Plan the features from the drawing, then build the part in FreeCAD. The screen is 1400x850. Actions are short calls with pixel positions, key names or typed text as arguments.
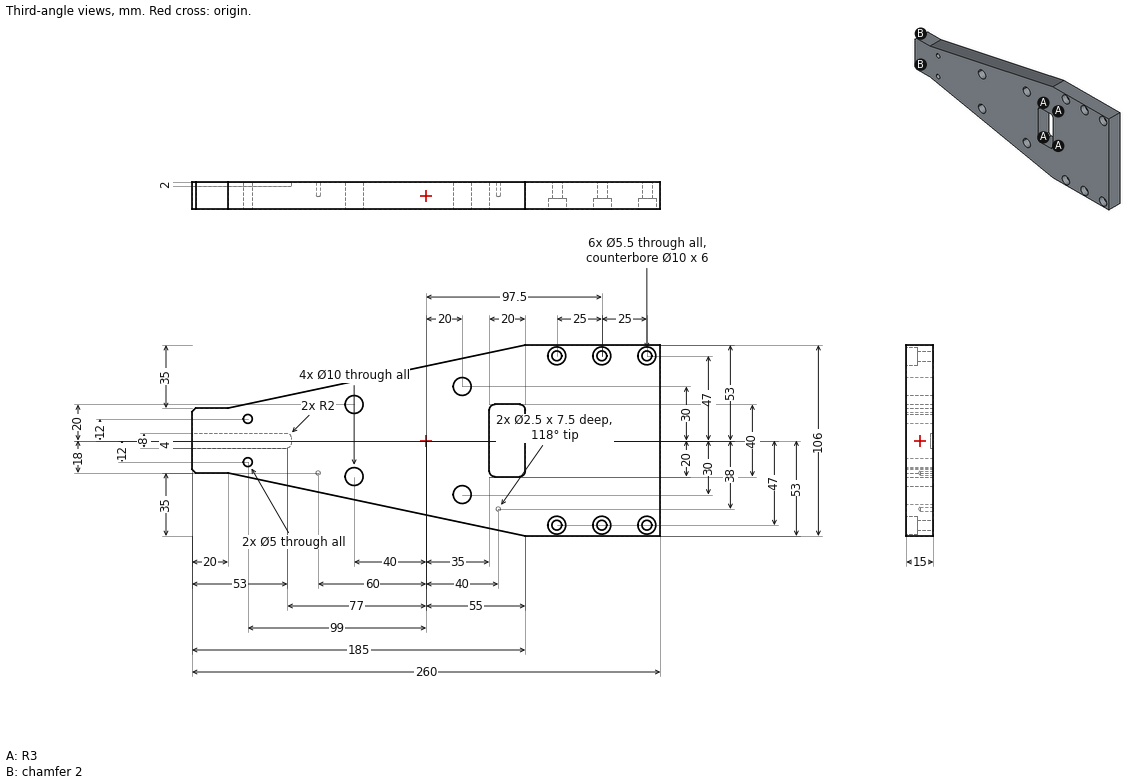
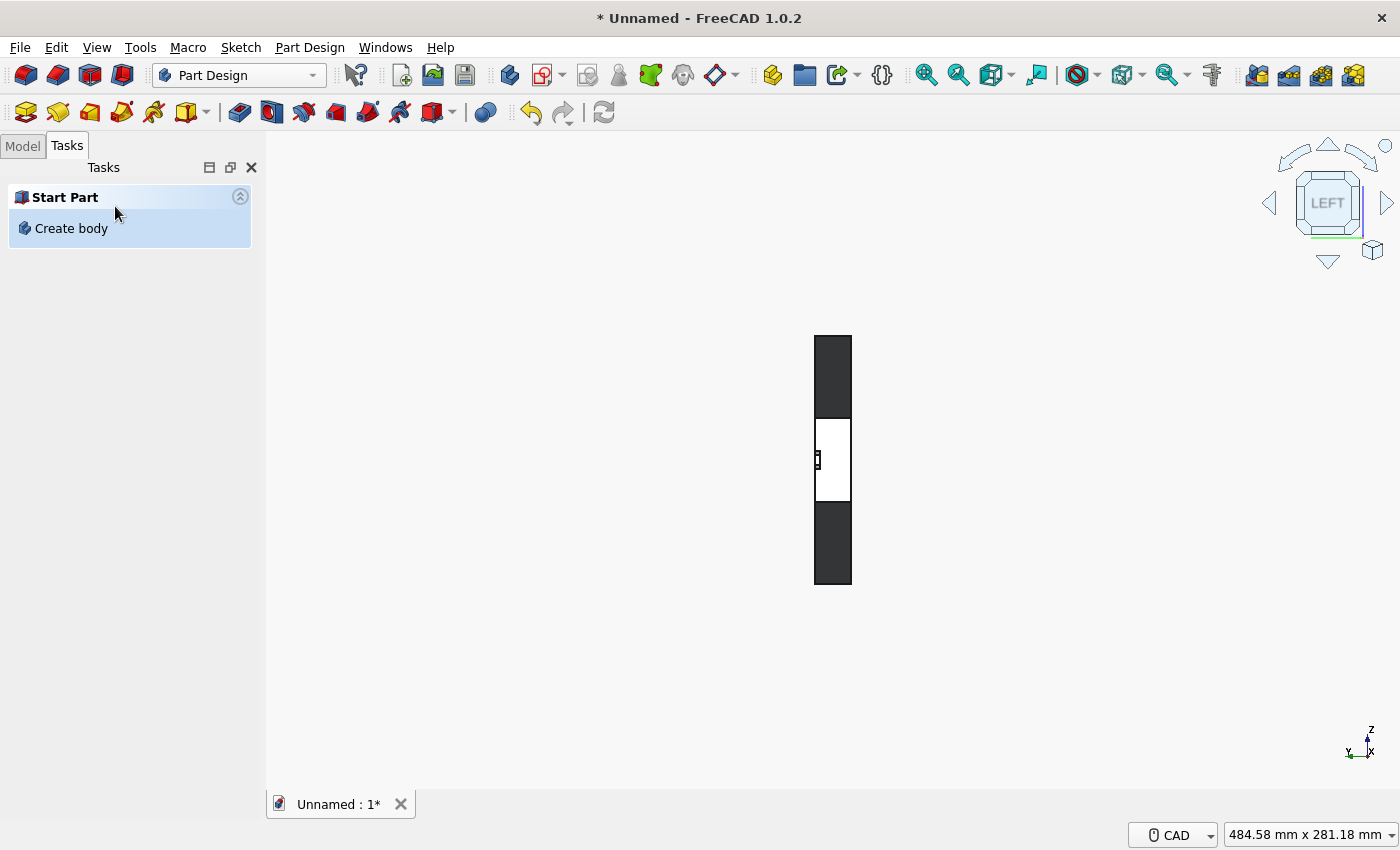
key(v)
key(3)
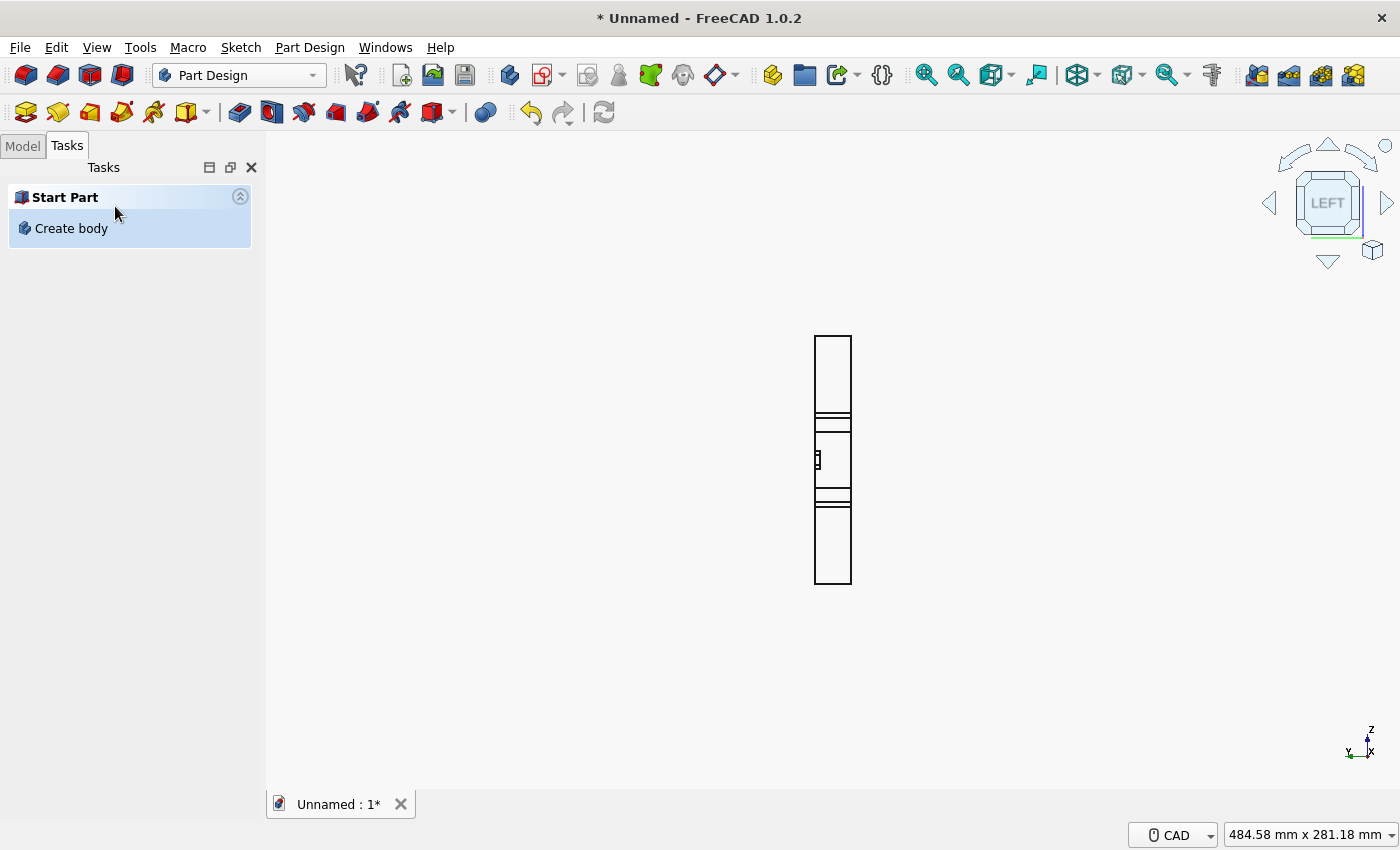
key(0)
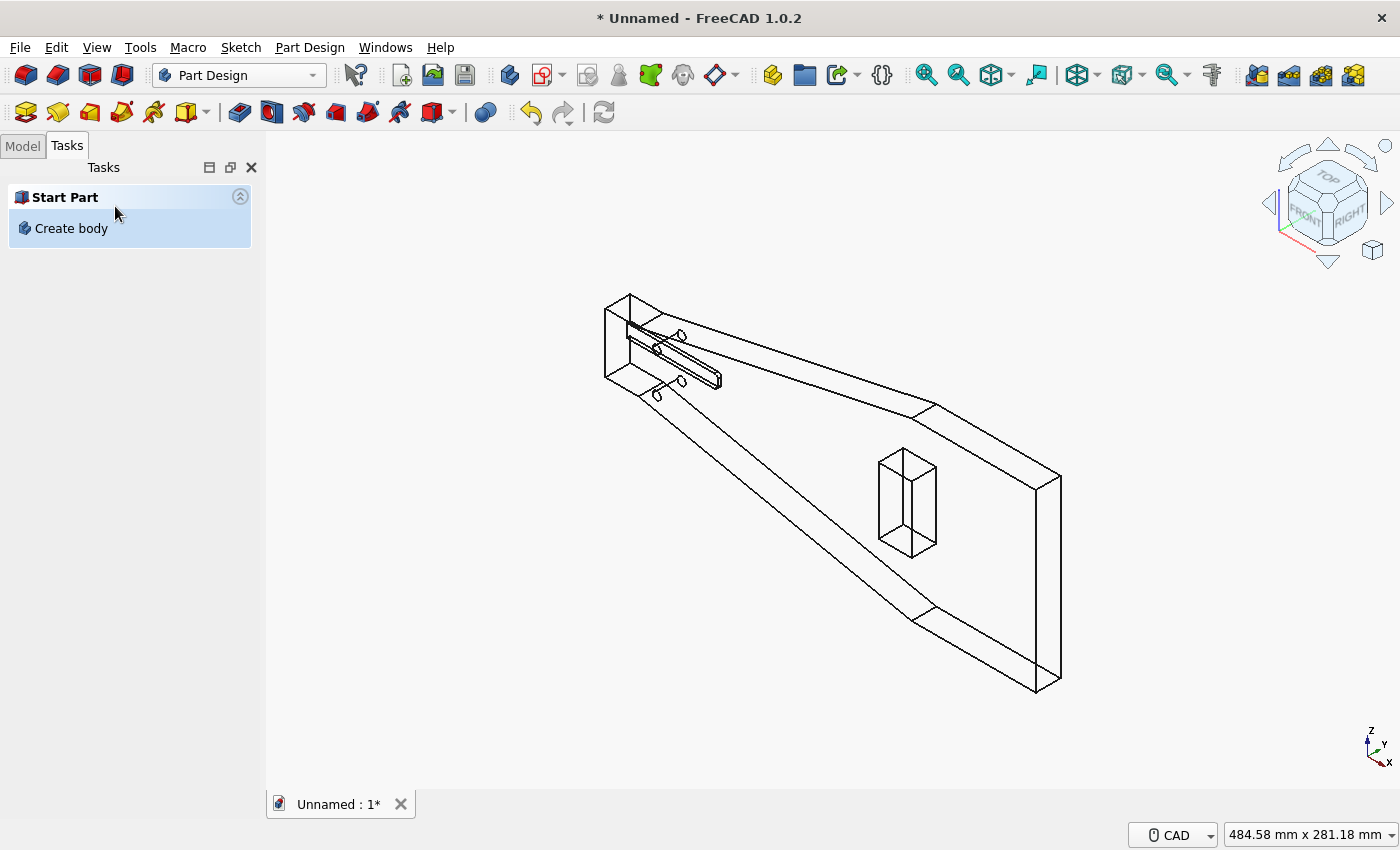
click(924, 550)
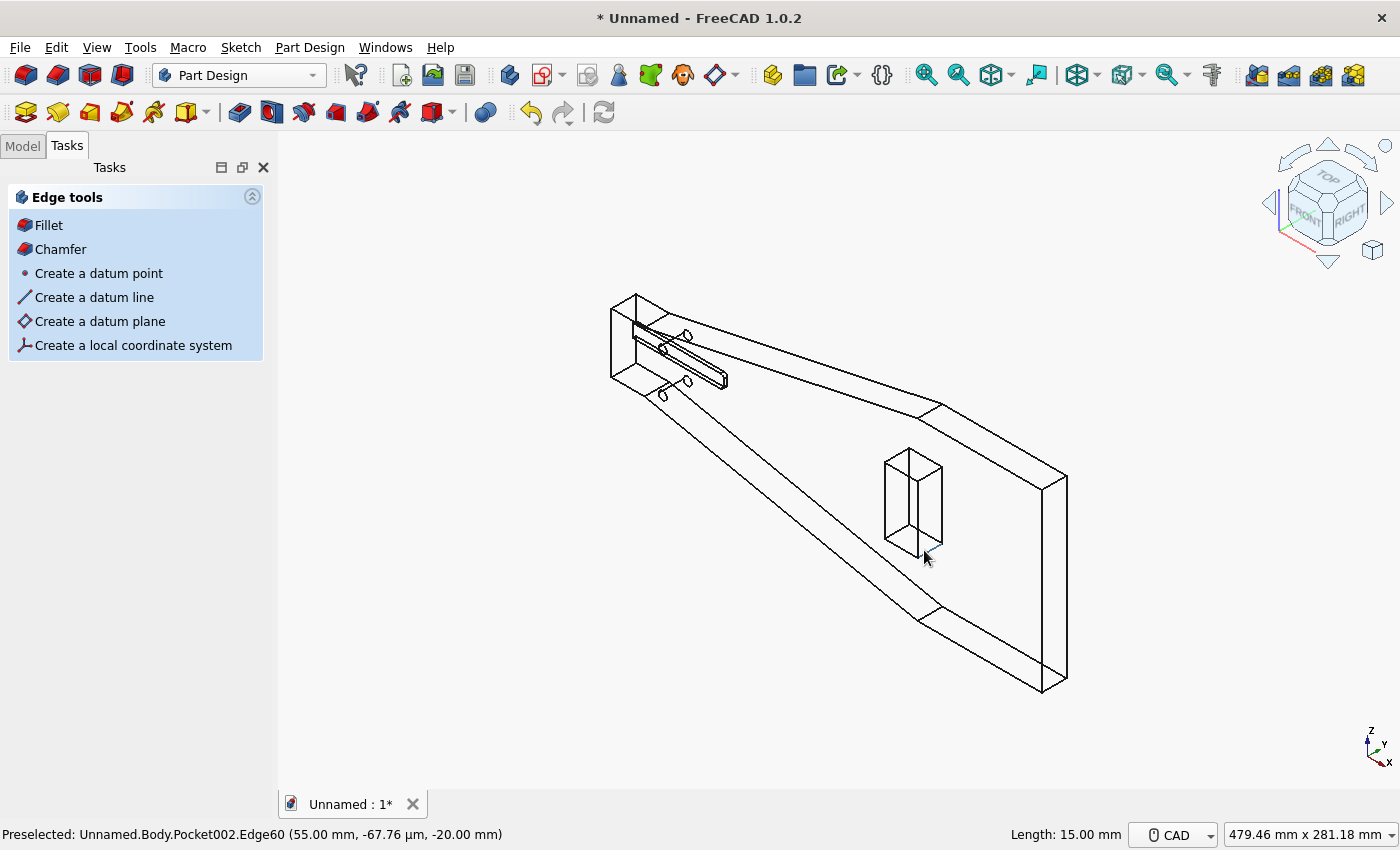
click(930, 473, ctrl)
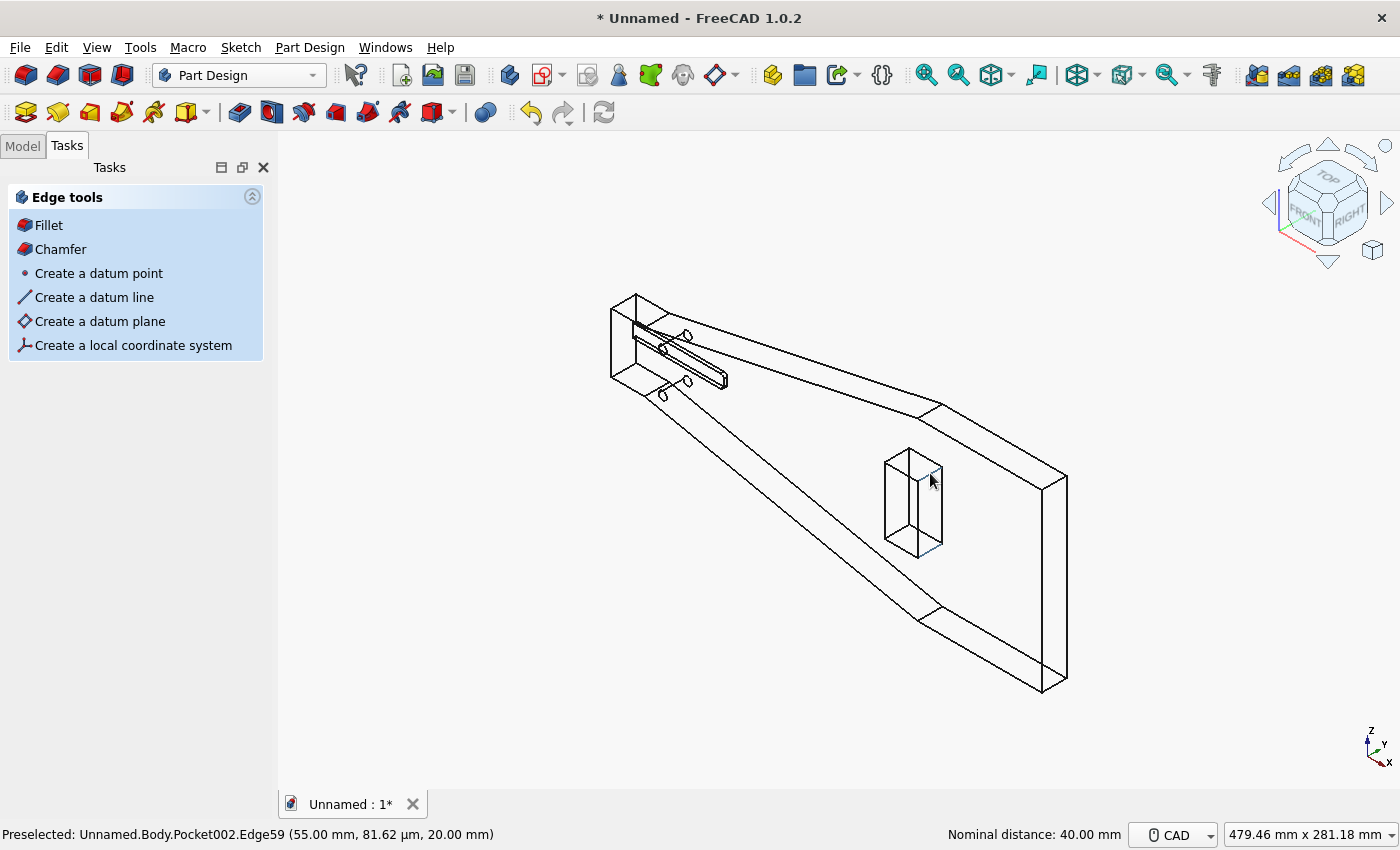
click(897, 454, ctrl)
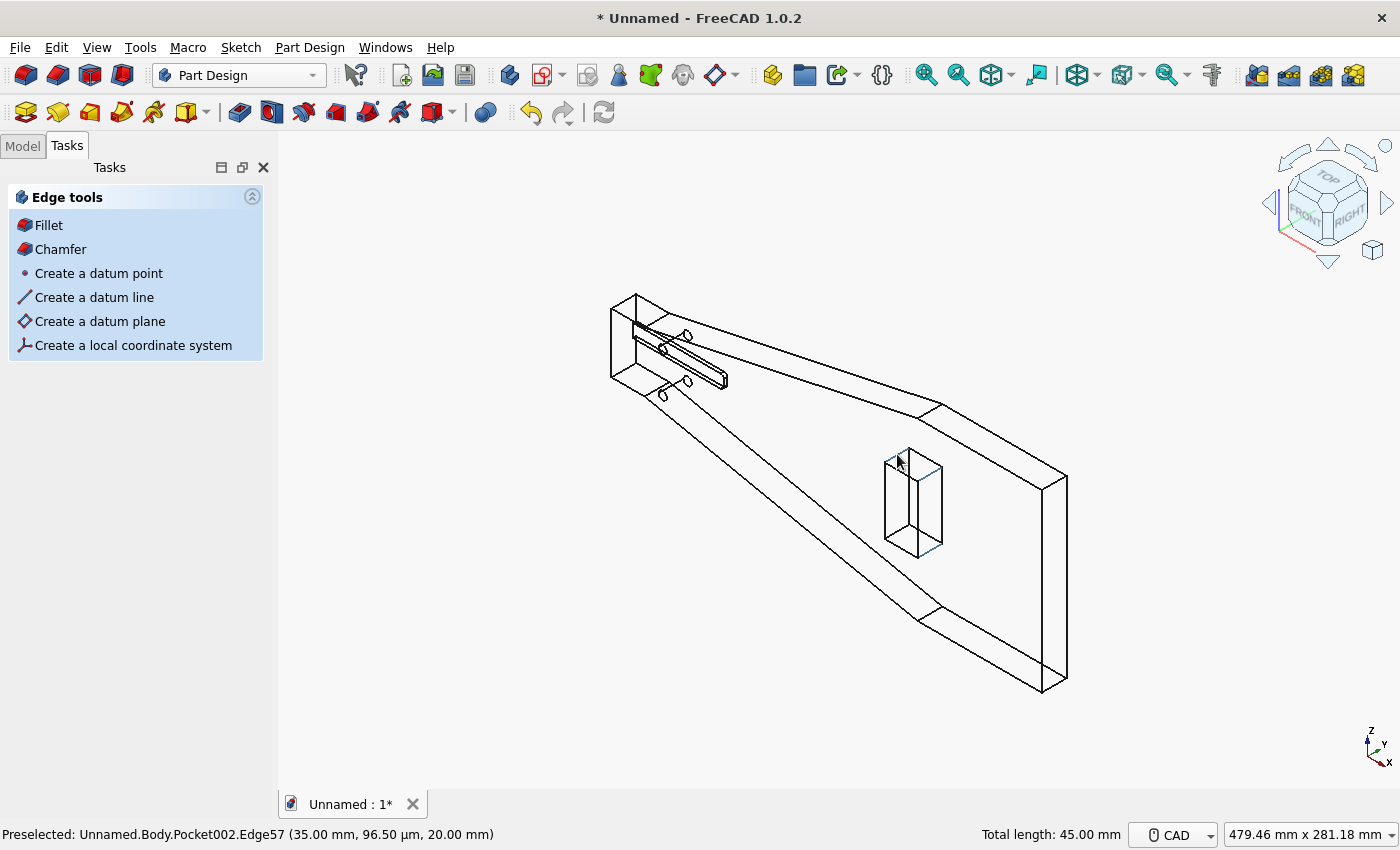
click(897, 531, ctrl)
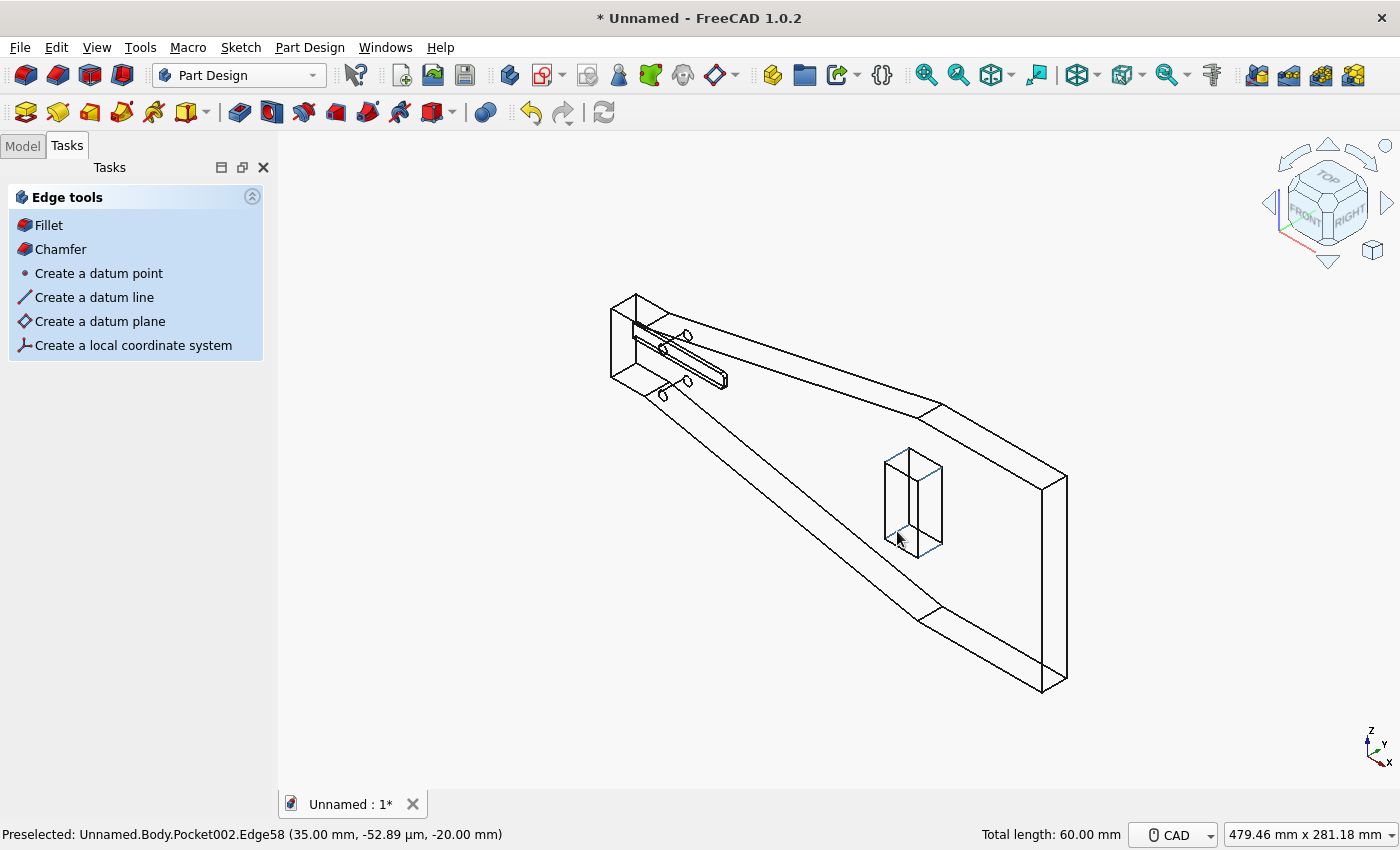
key(v)
key(1)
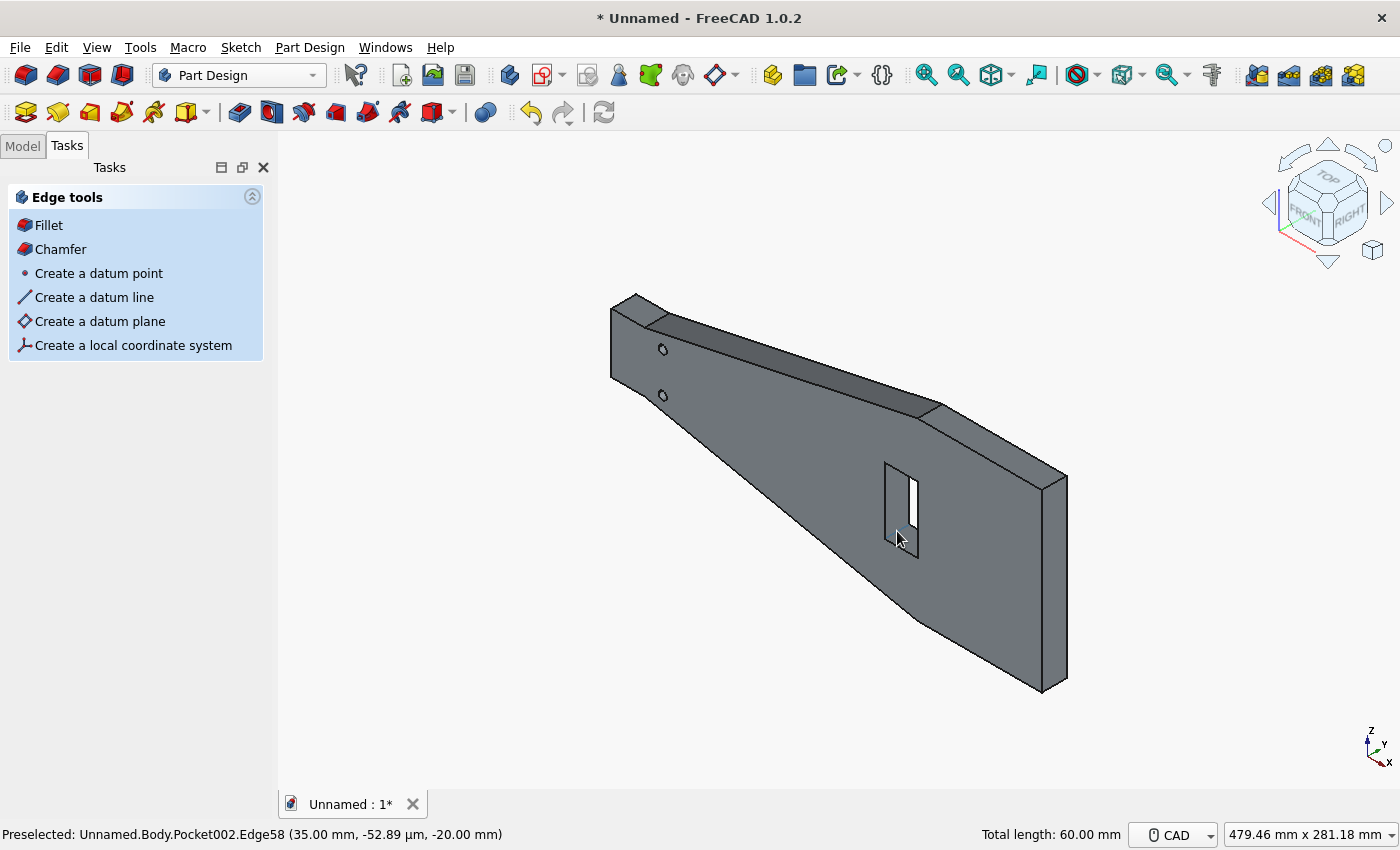
click(26, 76)